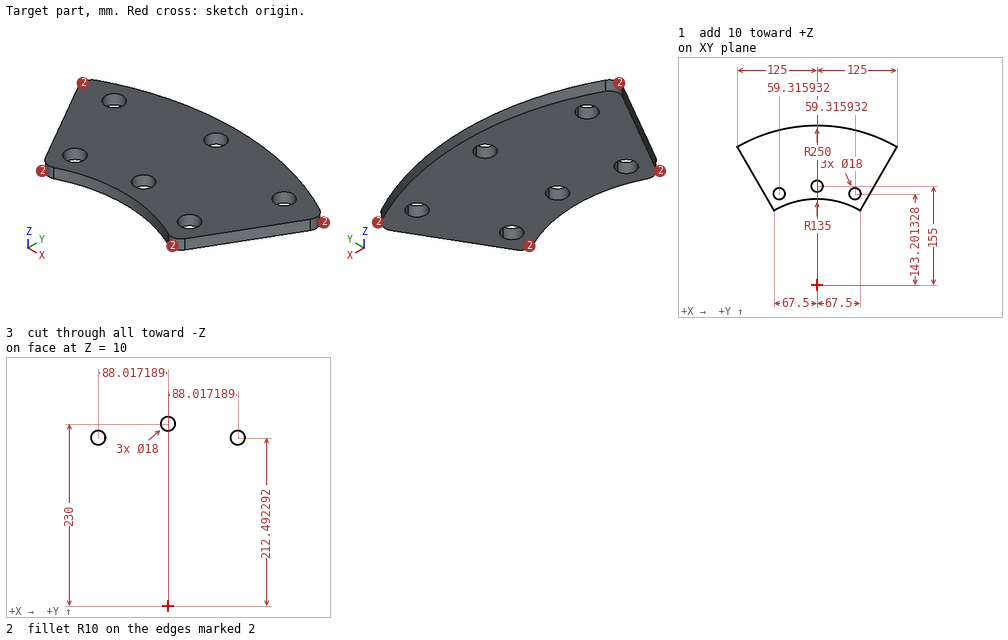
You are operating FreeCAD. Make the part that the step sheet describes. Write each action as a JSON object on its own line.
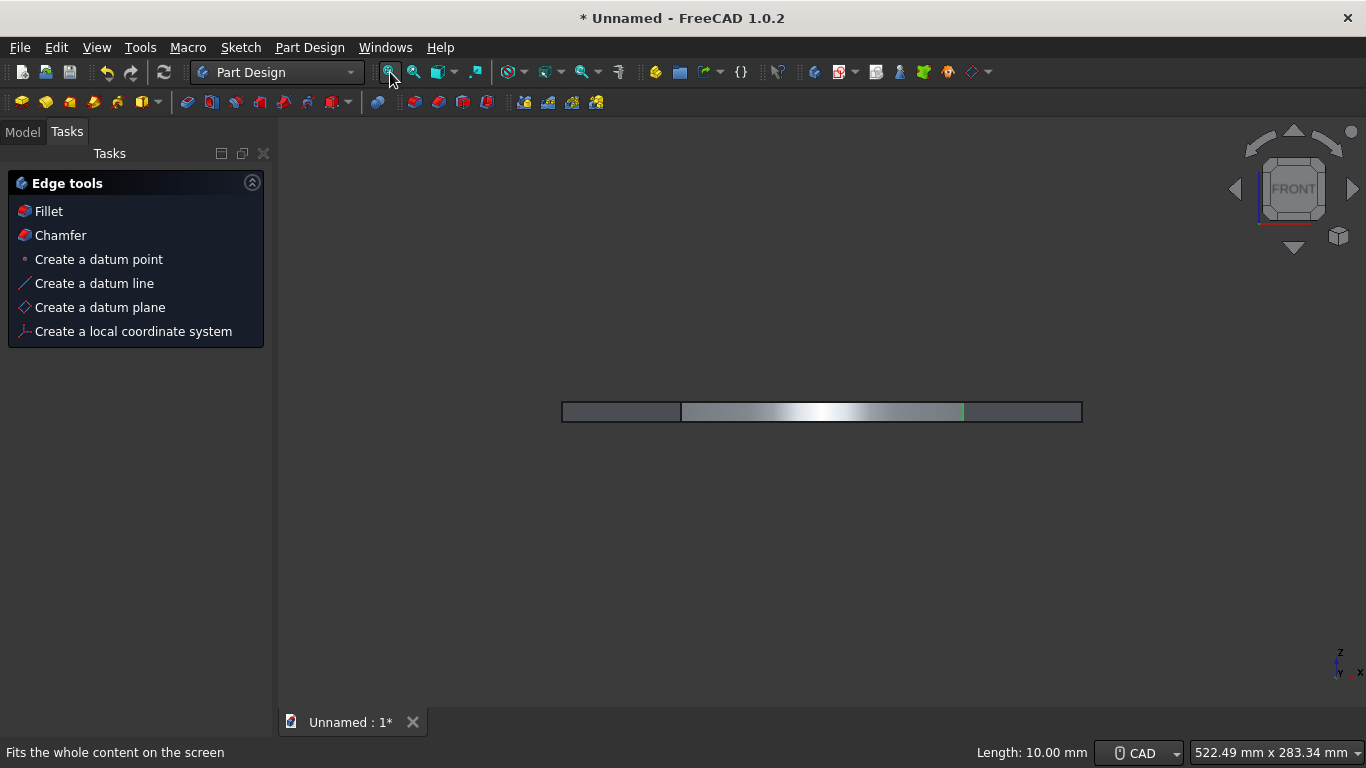
{"action": "left_click", "coordinate": [681, 411], "text": "ctrl"}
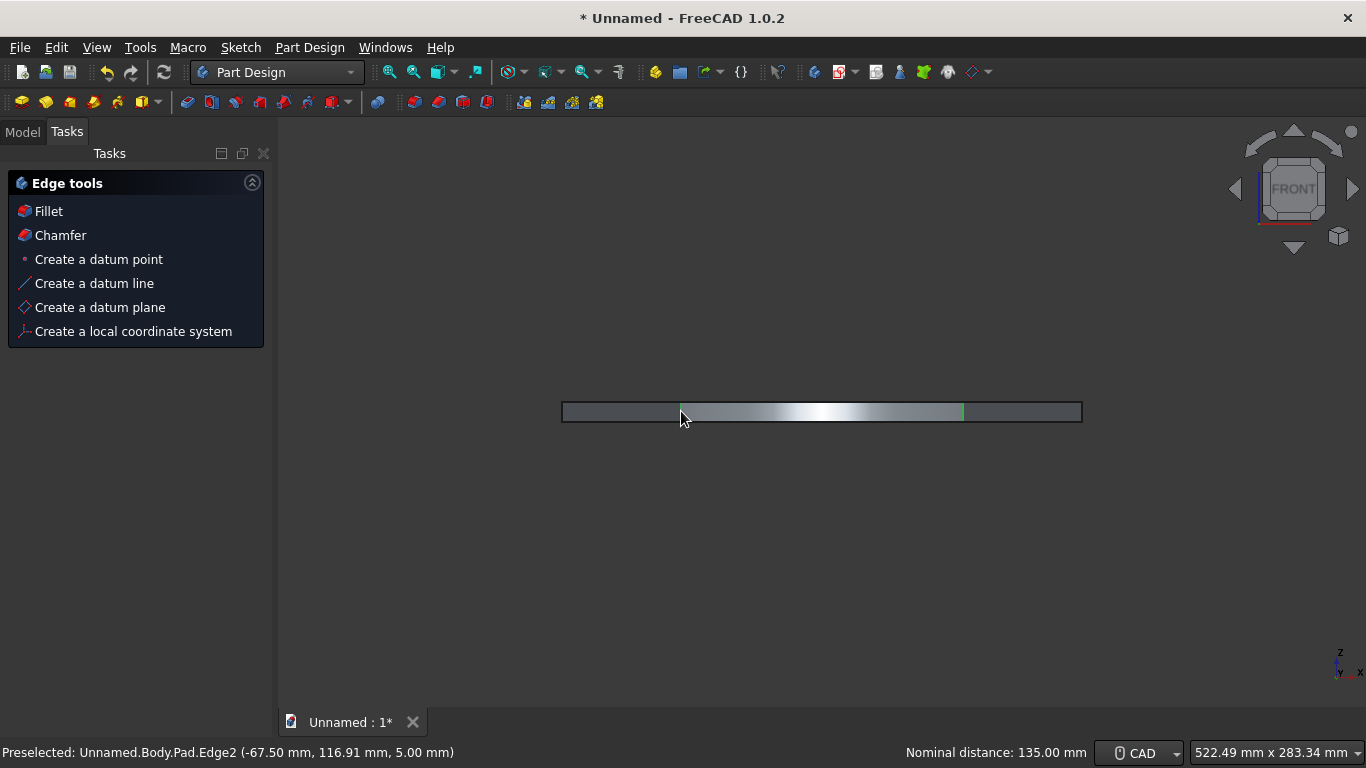
{"action": "scroll", "coordinate": [562, 411], "scroll_direction": "up", "scroll_amount": 4}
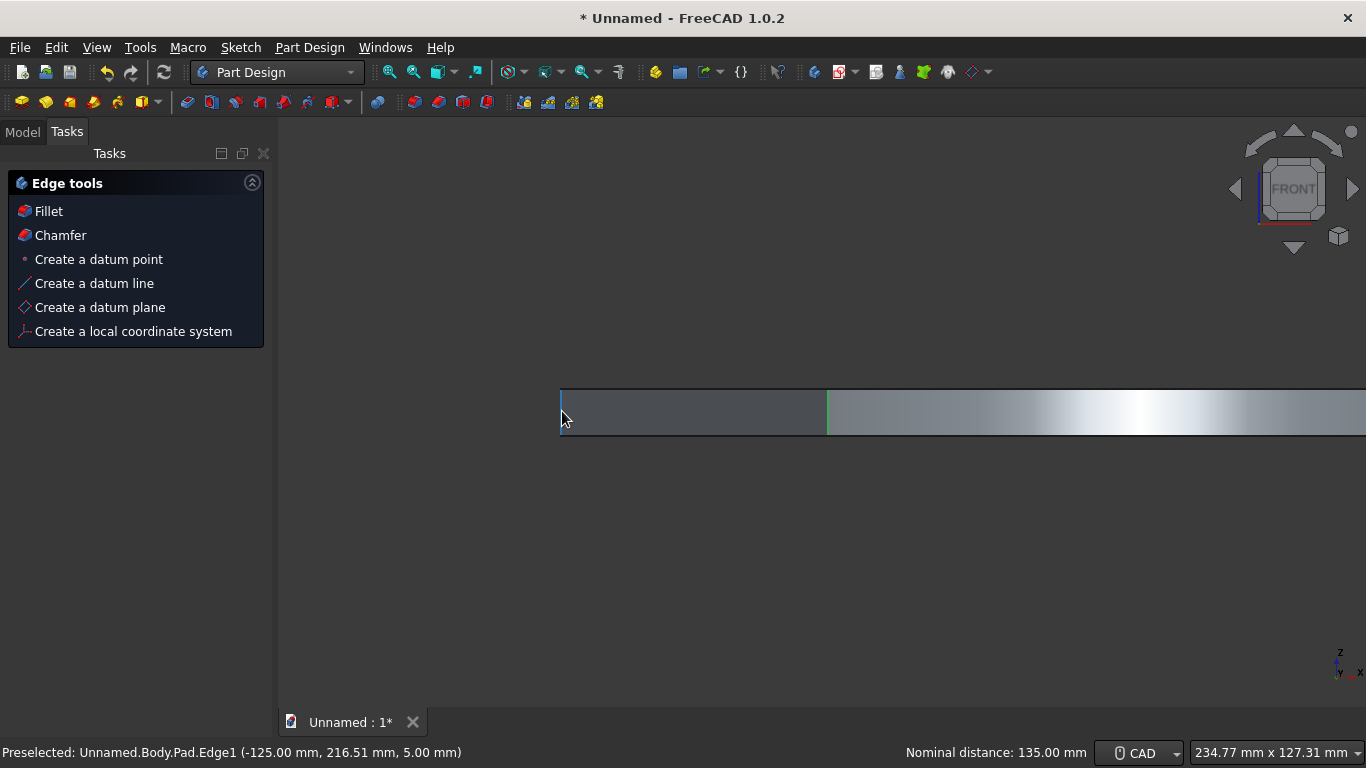
{"action": "key", "text": "v f"}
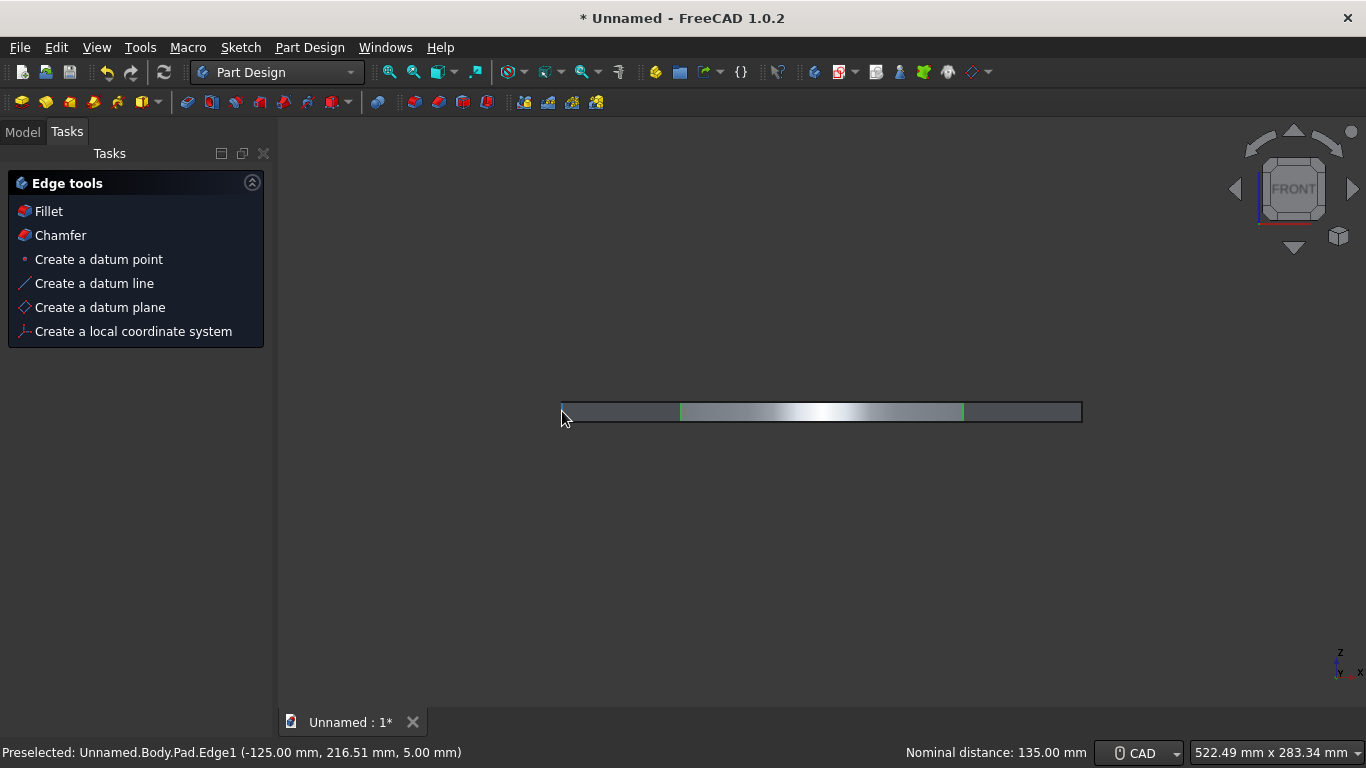
{"action": "key", "text": "3"}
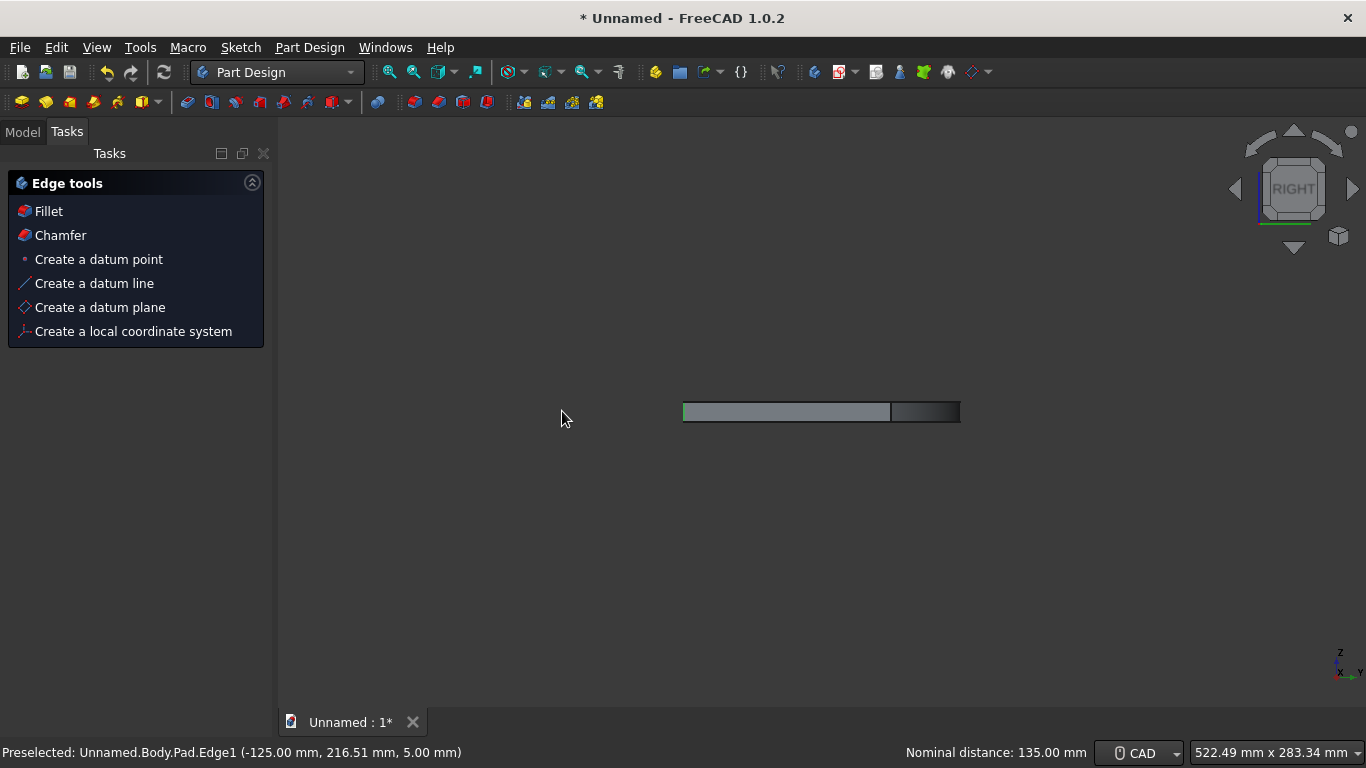
{"action": "left_click", "coordinate": [390, 72]}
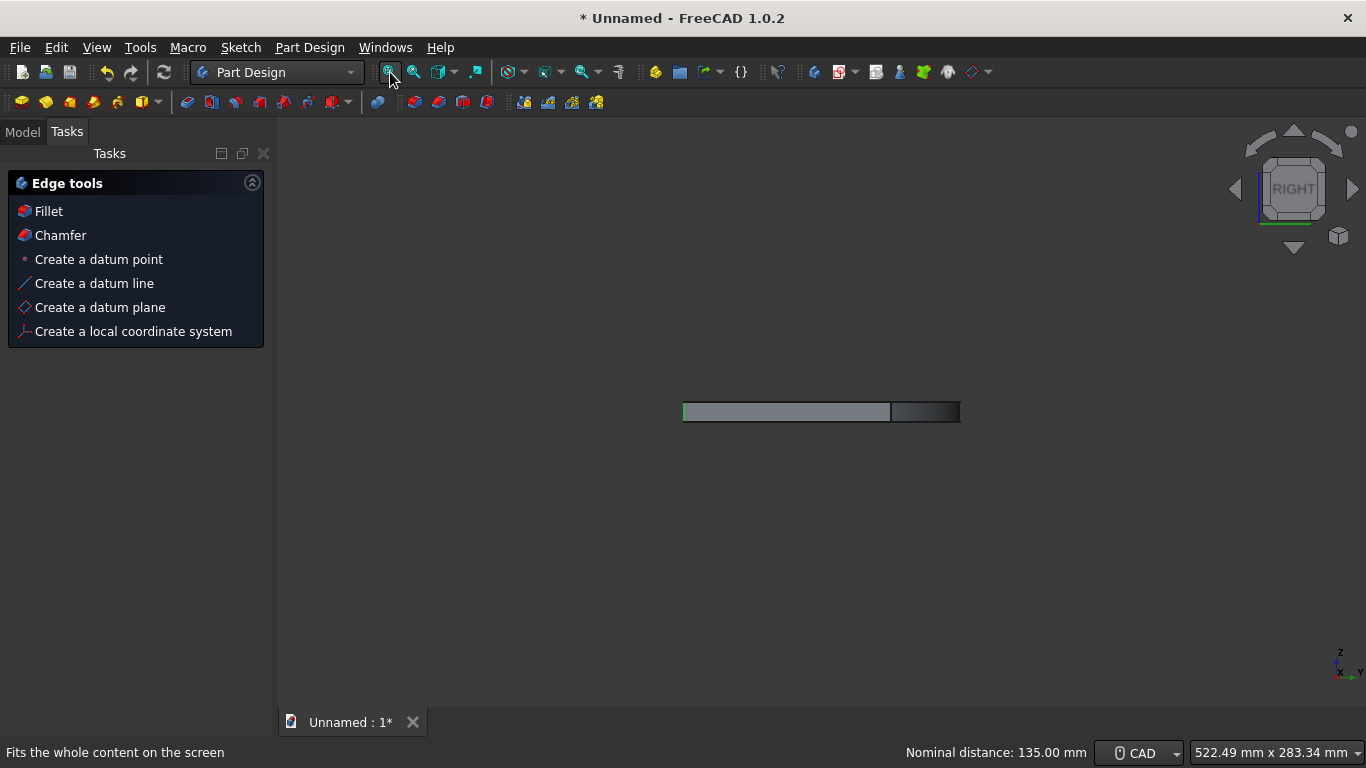
{"action": "left_click", "coordinate": [891, 411], "text": "ctrl"}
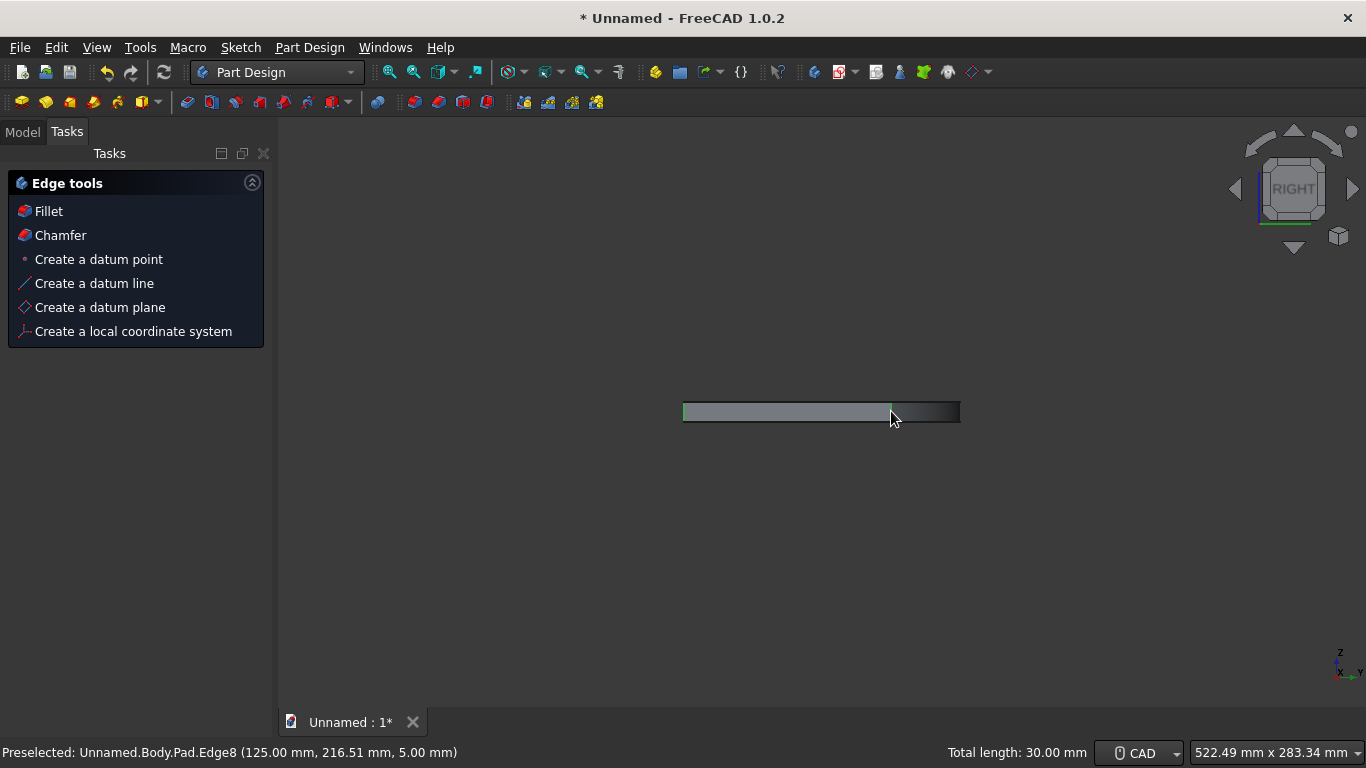
{"action": "scroll", "coordinate": [891, 411], "scroll_direction": "up", "scroll_amount": 4}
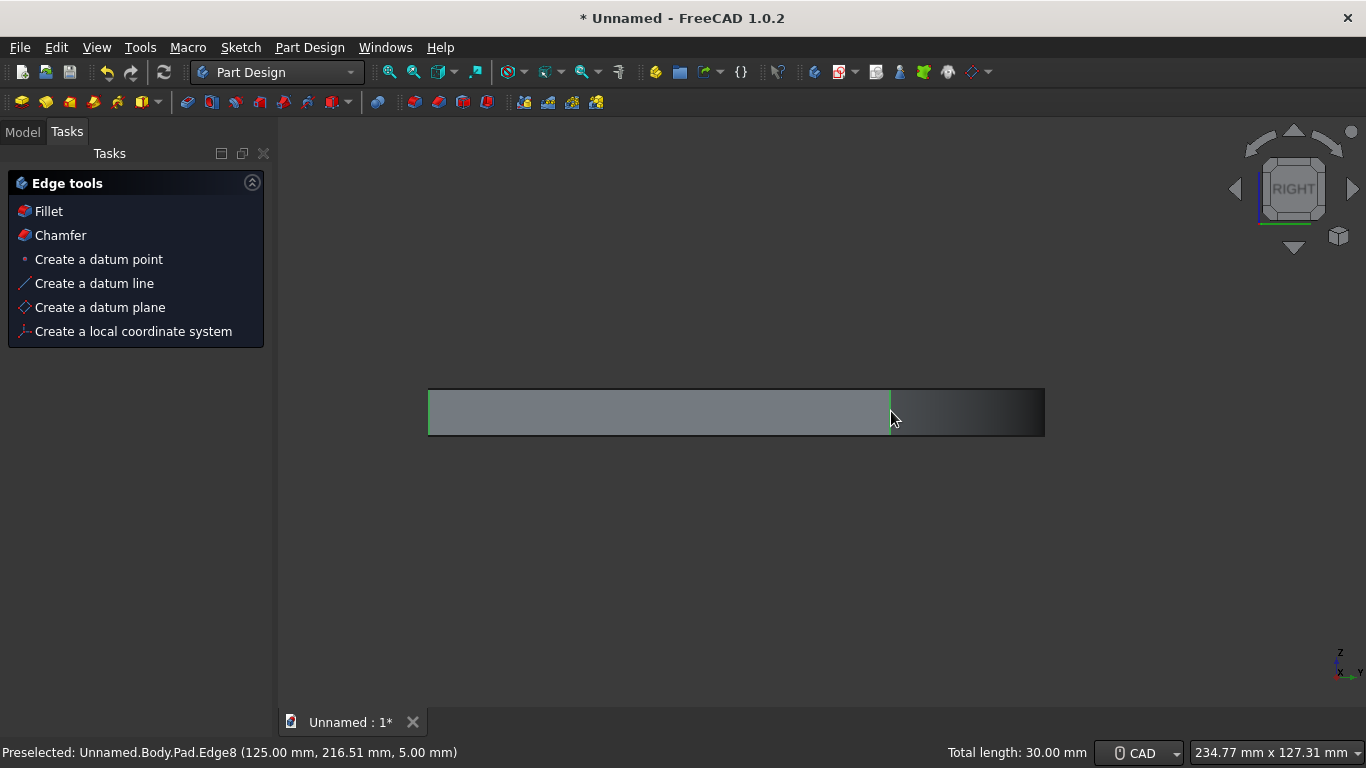
{"action": "left_click", "coordinate": [390, 72]}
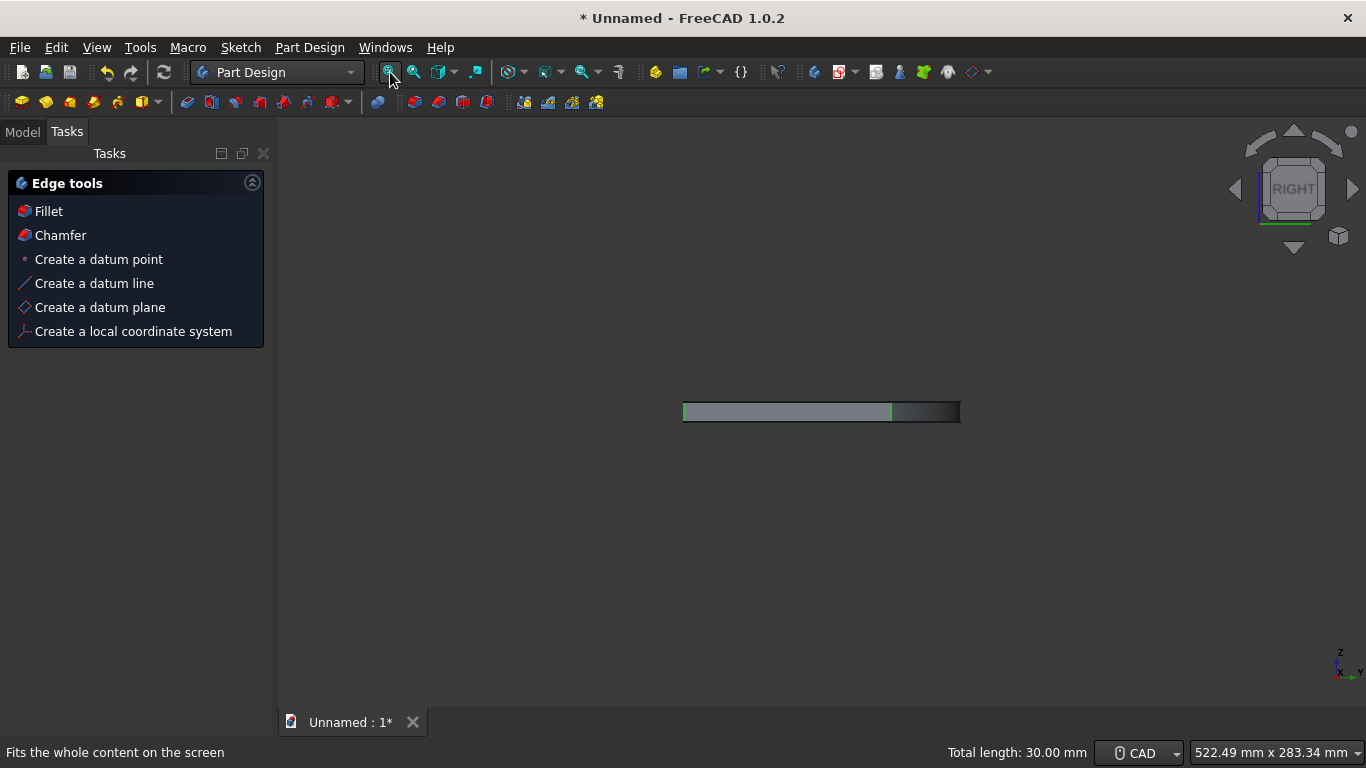
{"action": "key", "text": "5"}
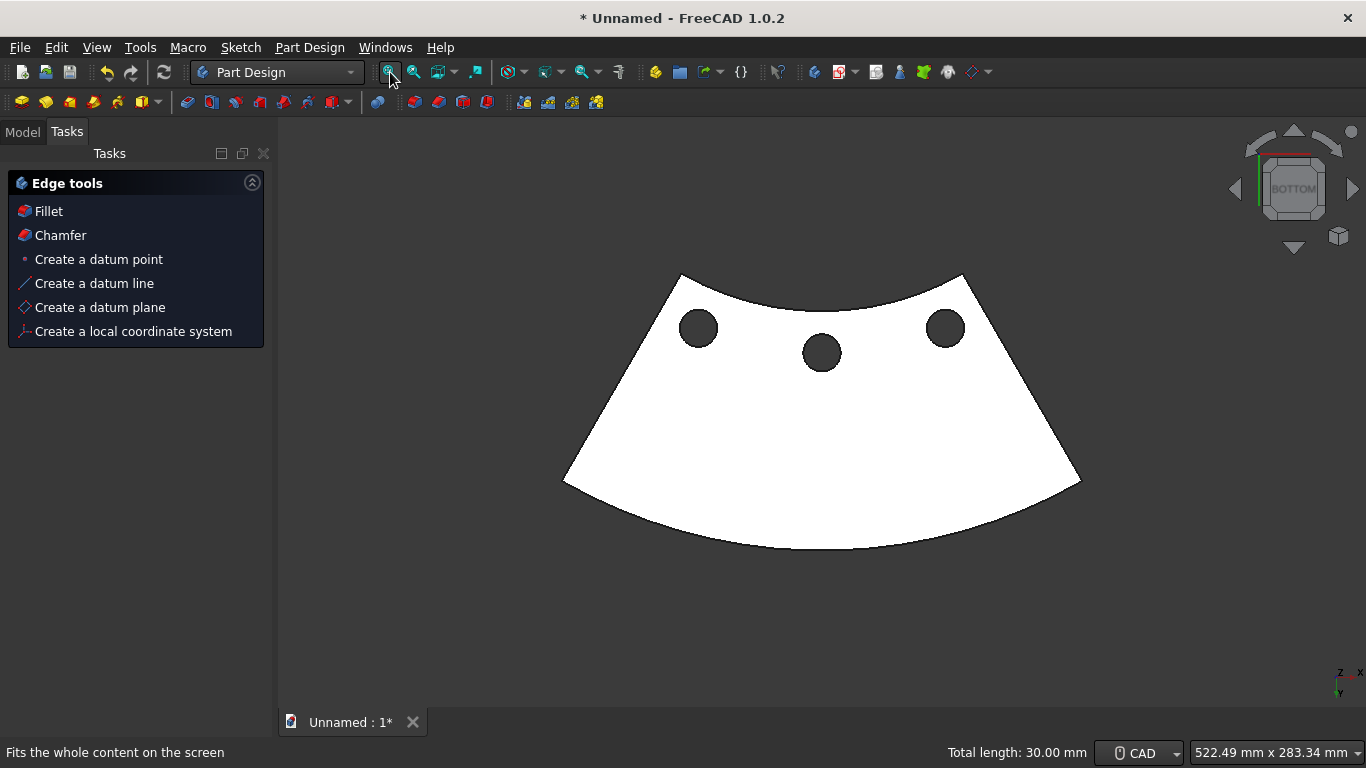
{"action": "scroll", "coordinate": [562, 480], "scroll_direction": "up", "scroll_amount": 4}